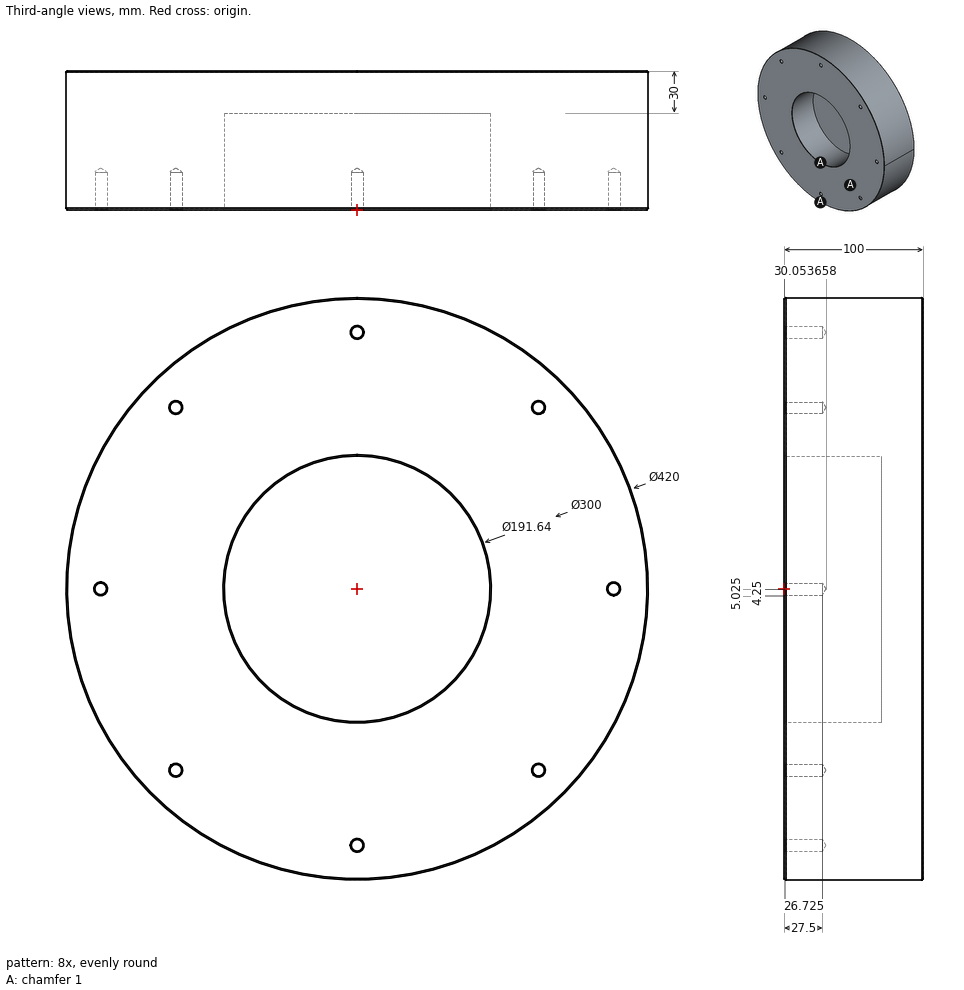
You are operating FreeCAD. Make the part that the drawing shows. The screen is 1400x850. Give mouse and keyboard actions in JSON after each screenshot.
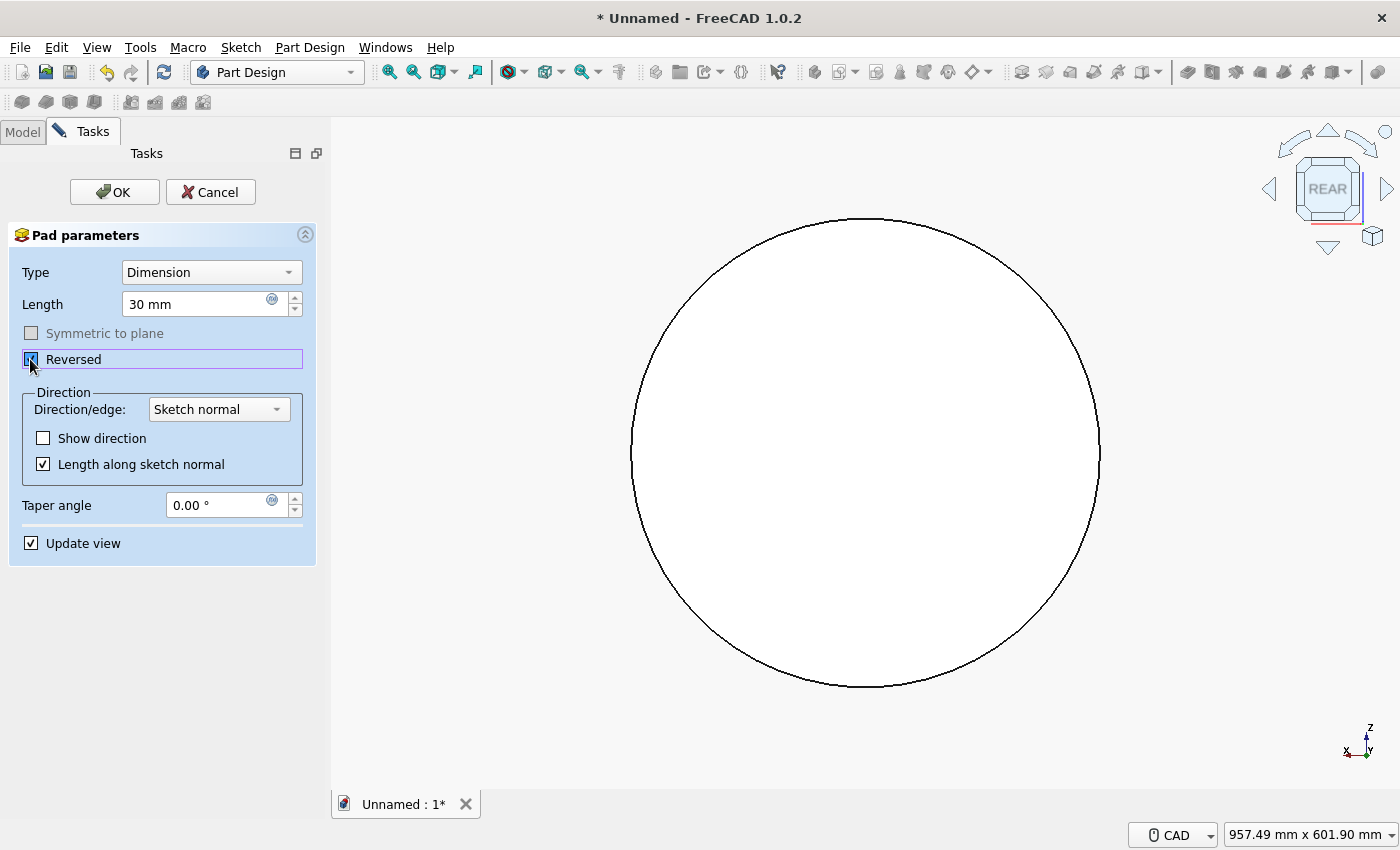
{"action": "left_click", "coordinate": [115, 192]}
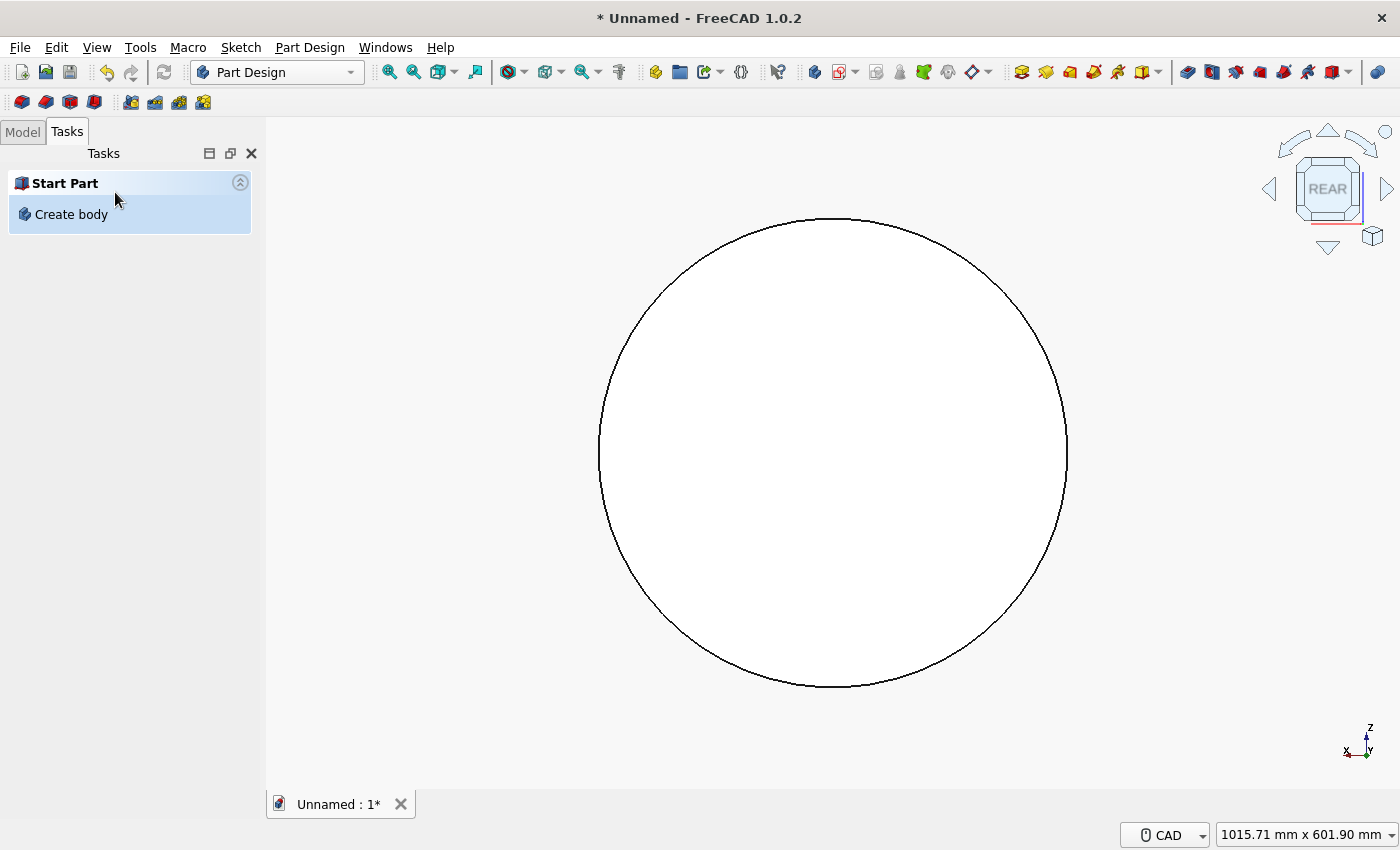
{"action": "left_click", "coordinate": [23, 131]}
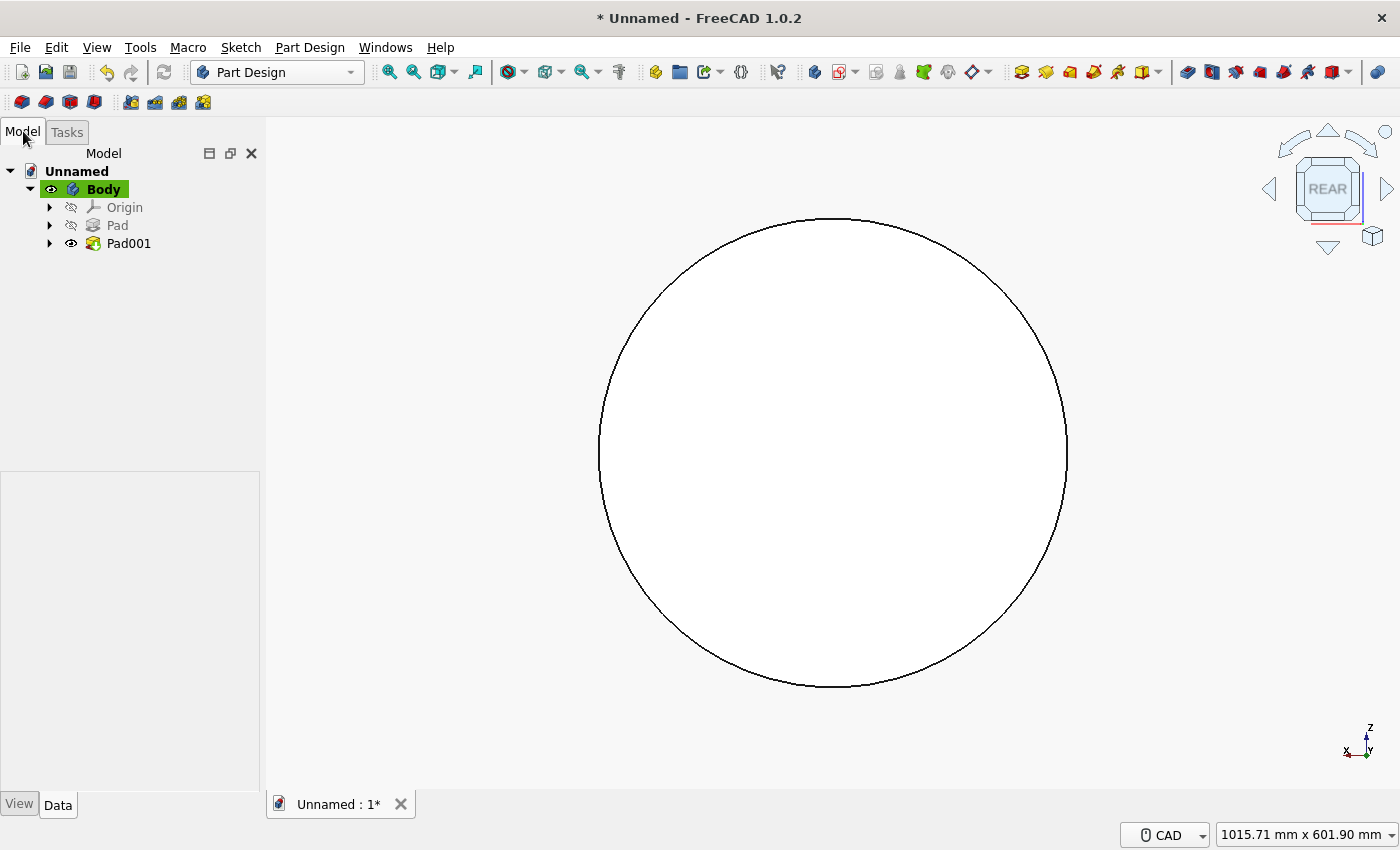
{"action": "left_click", "coordinate": [50, 207]}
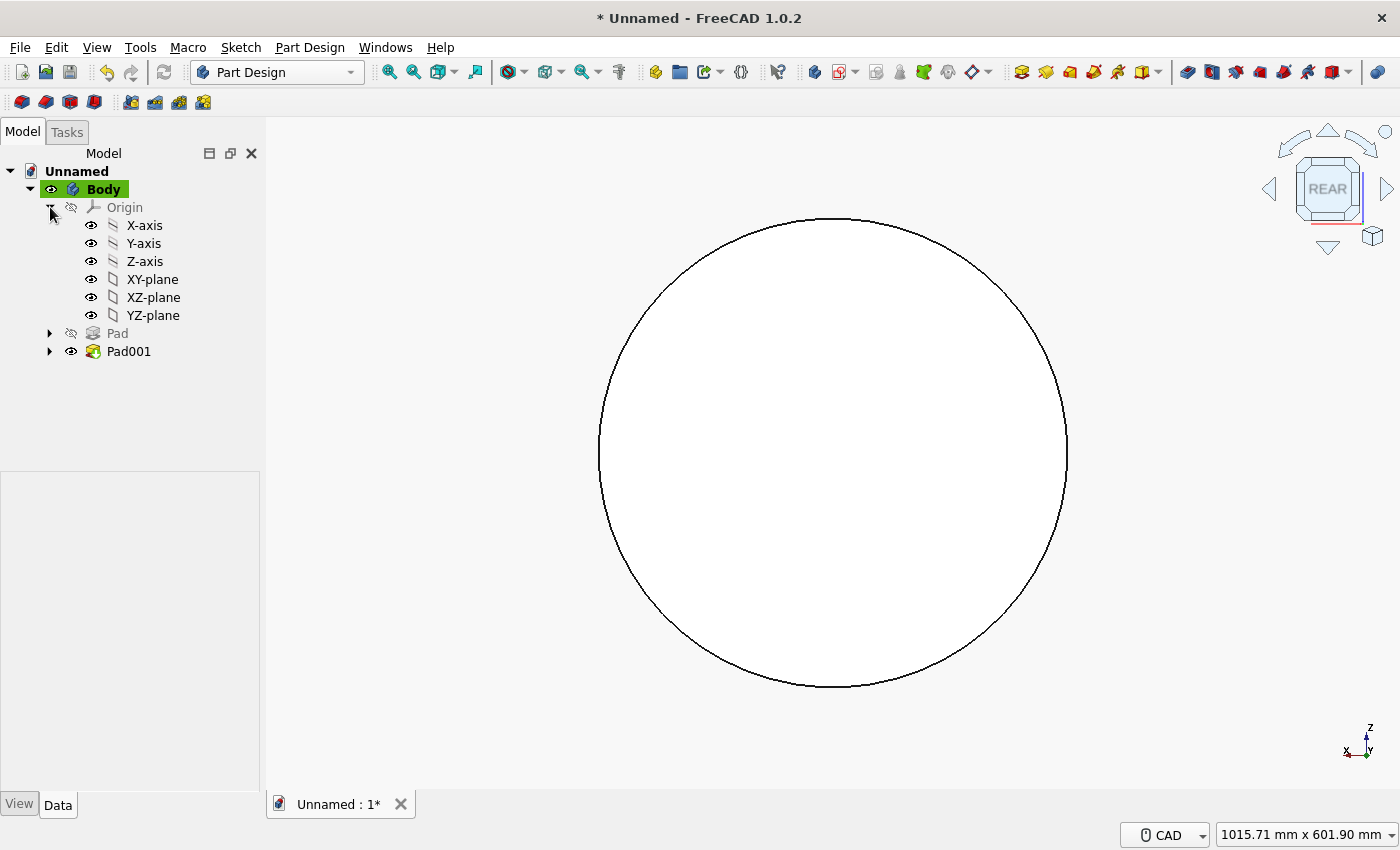
{"action": "left_click", "coordinate": [136, 315]}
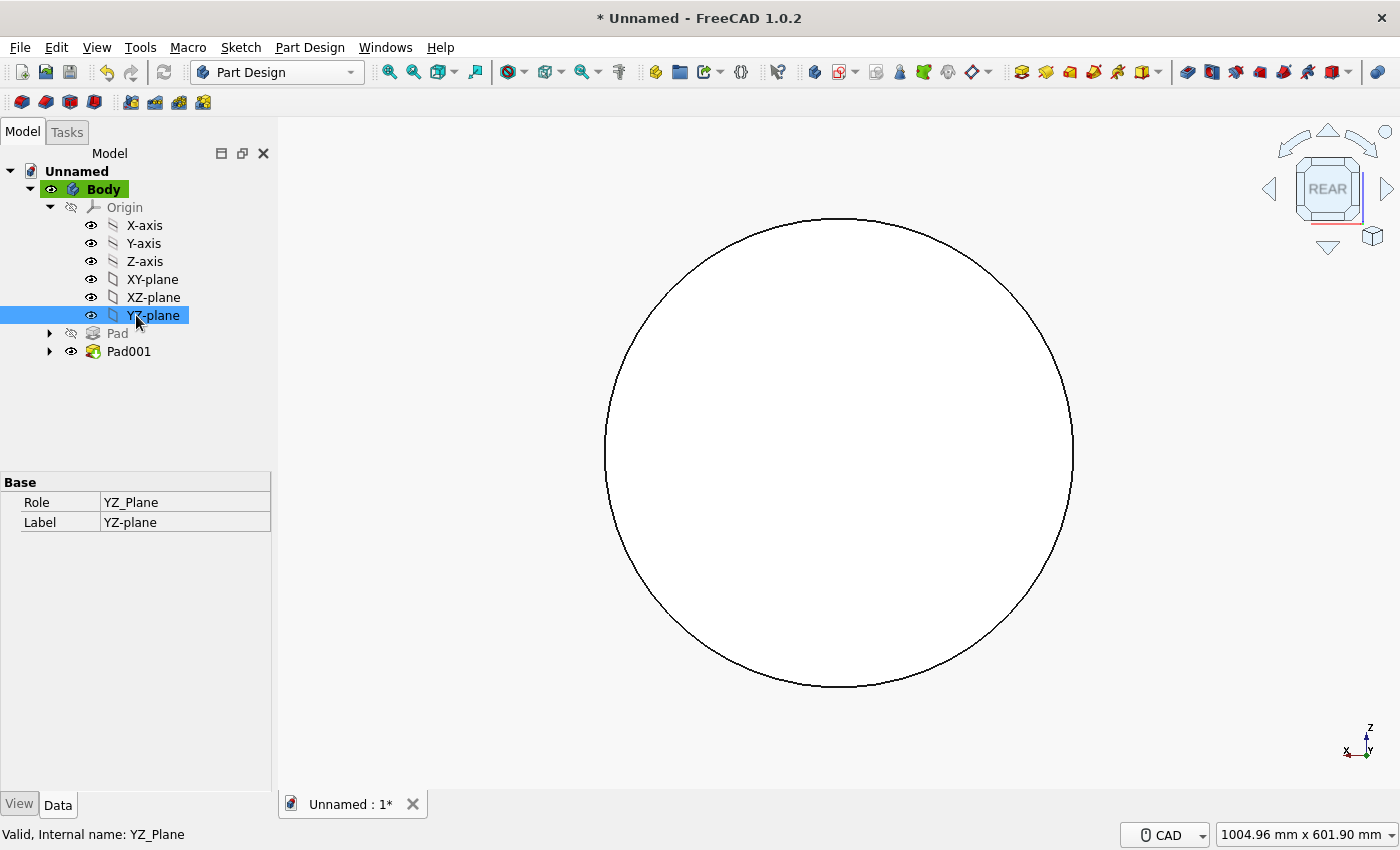
{"action": "left_click", "coordinate": [972, 72]}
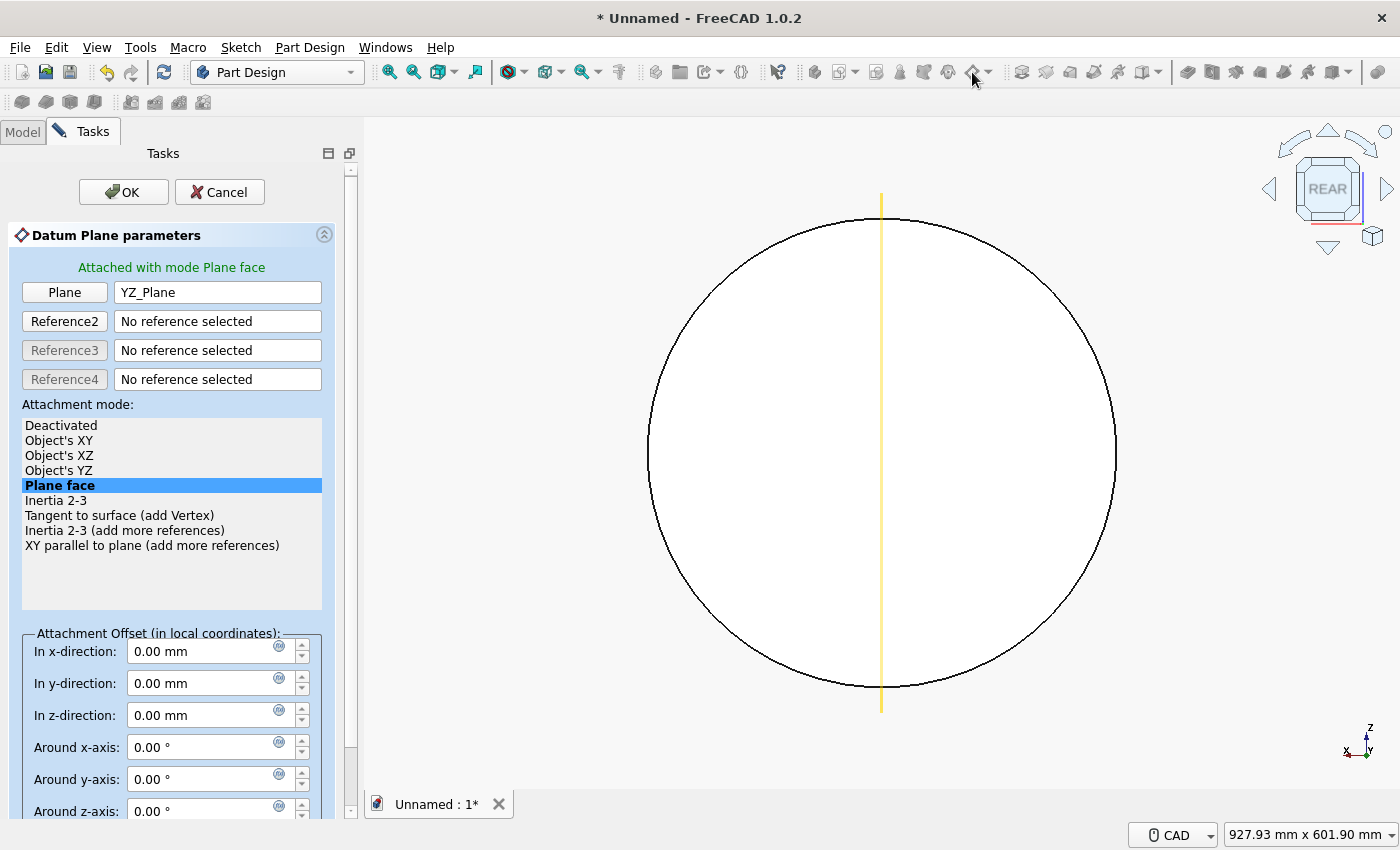
{"action": "triple_click", "coordinate": [210, 715]}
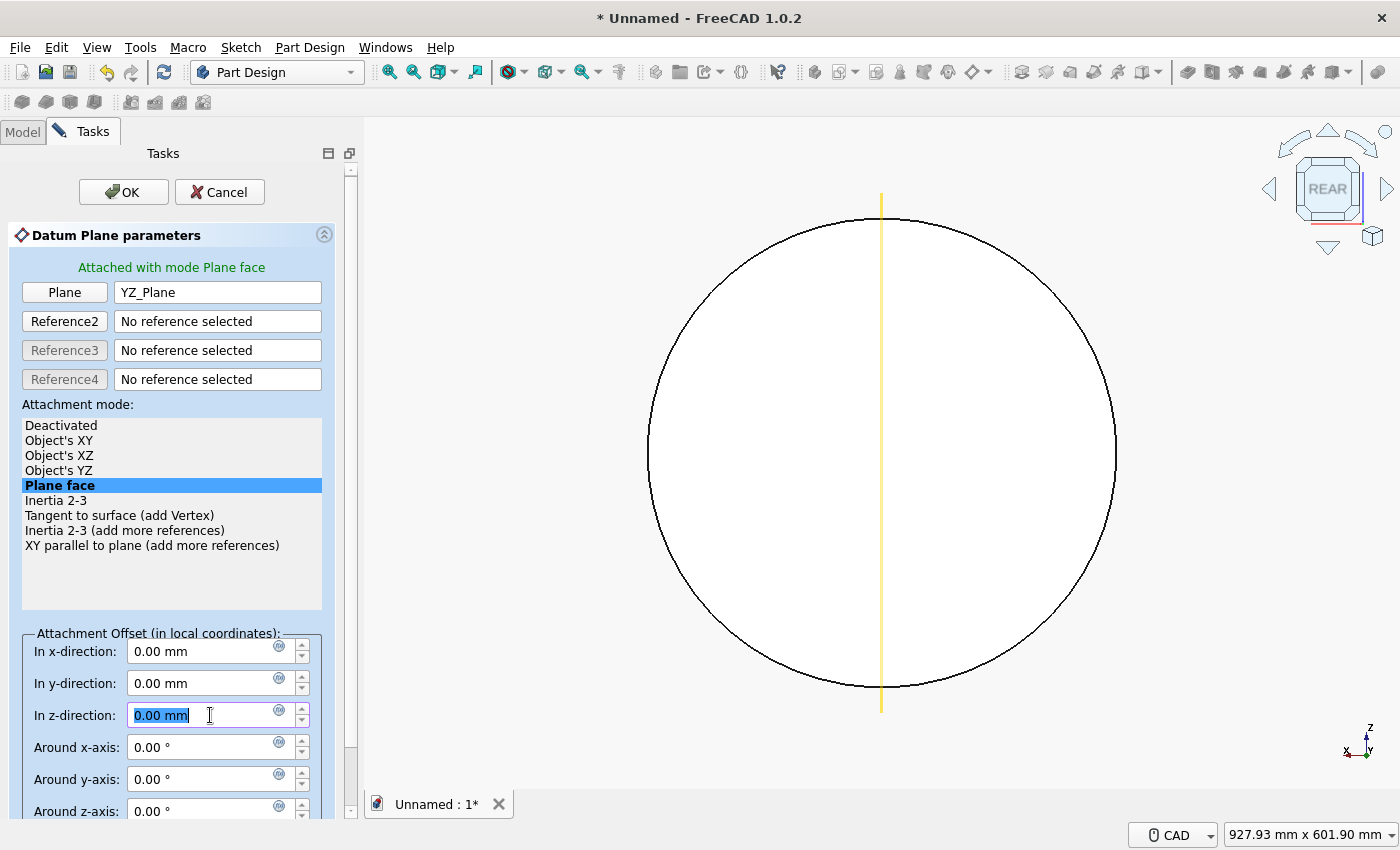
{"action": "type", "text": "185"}
{"action": "key", "text": "Tab"}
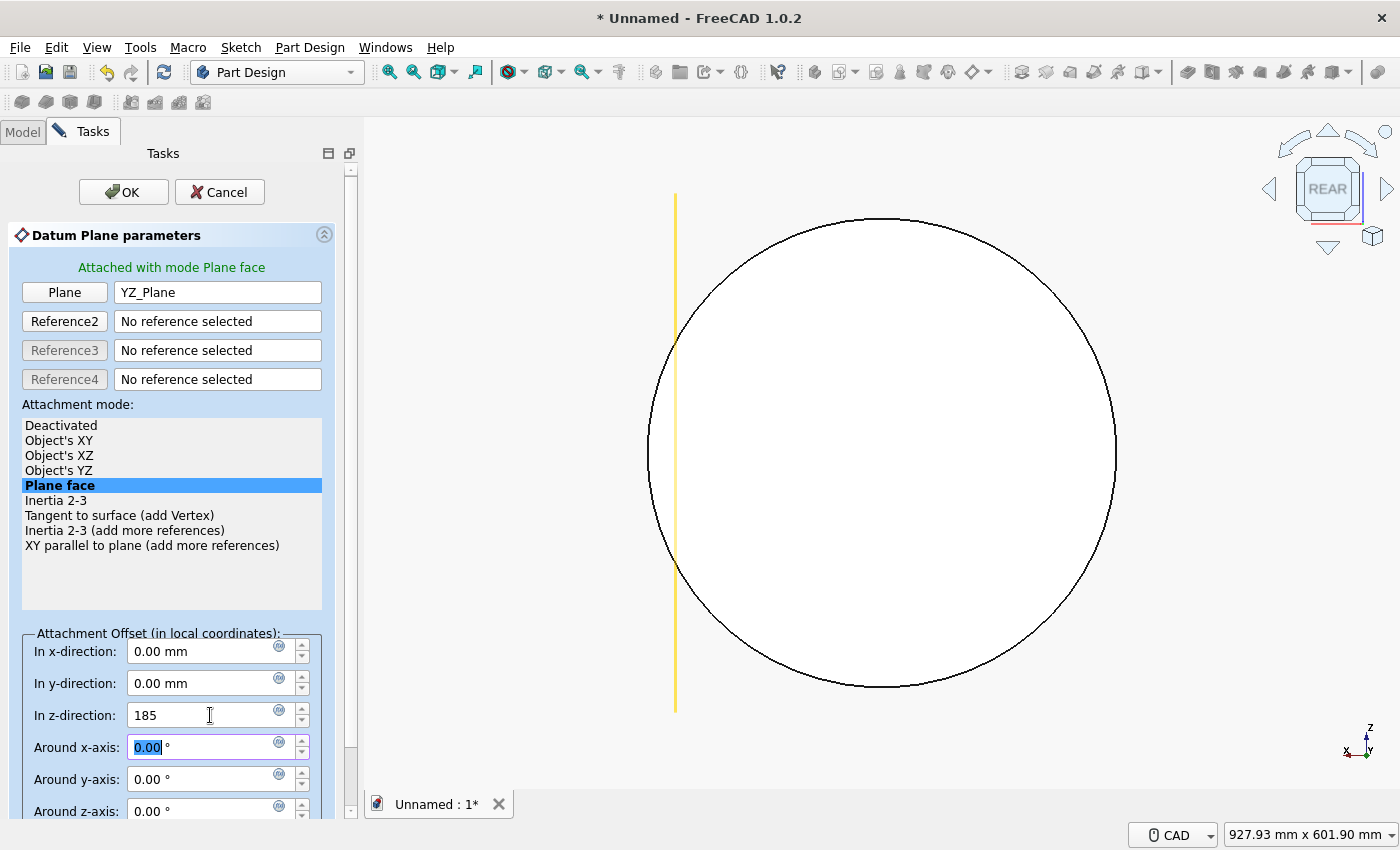
{"action": "left_click", "coordinate": [124, 192]}